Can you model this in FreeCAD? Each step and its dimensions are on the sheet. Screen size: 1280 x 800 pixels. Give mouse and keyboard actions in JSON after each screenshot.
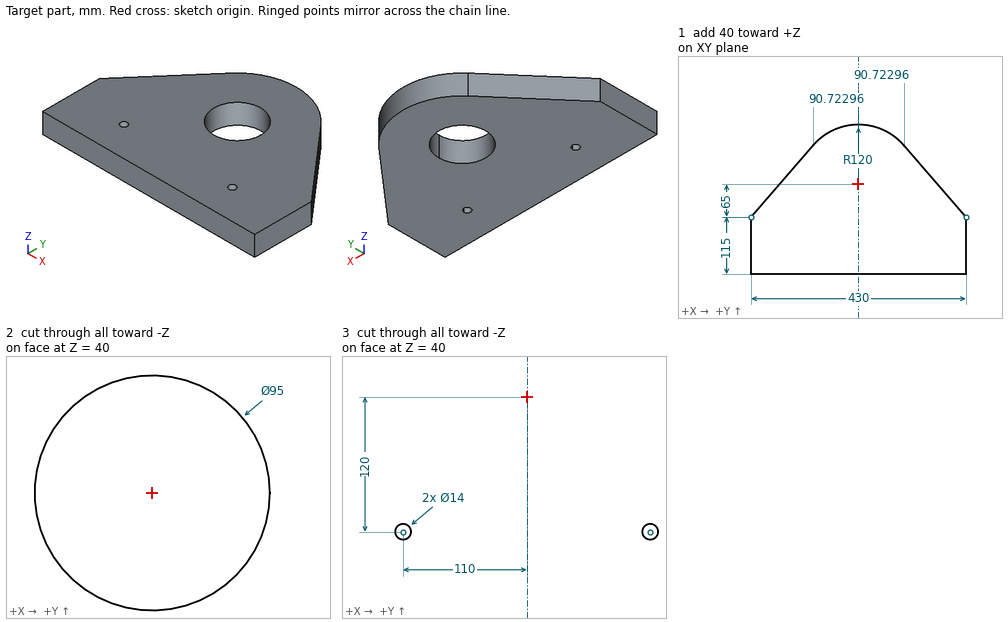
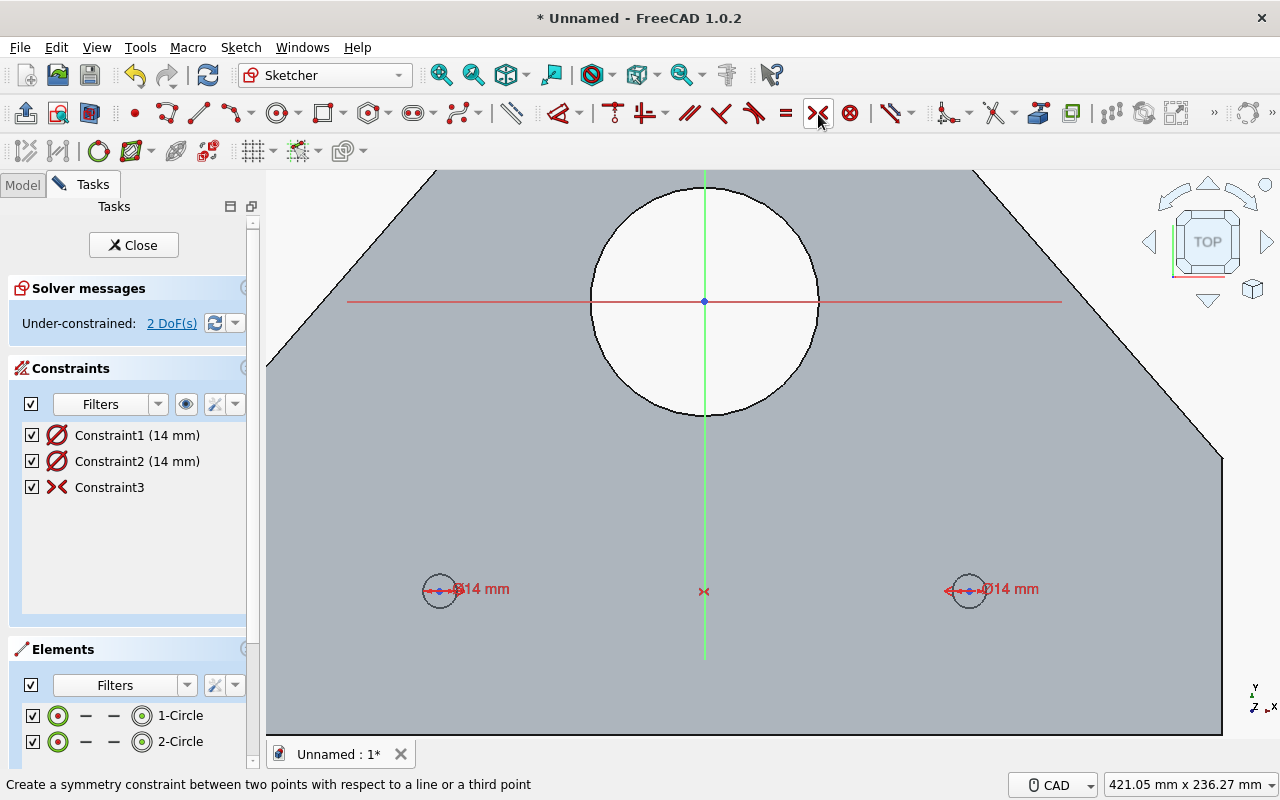
{"action": "left_click", "coordinate": [558, 114]}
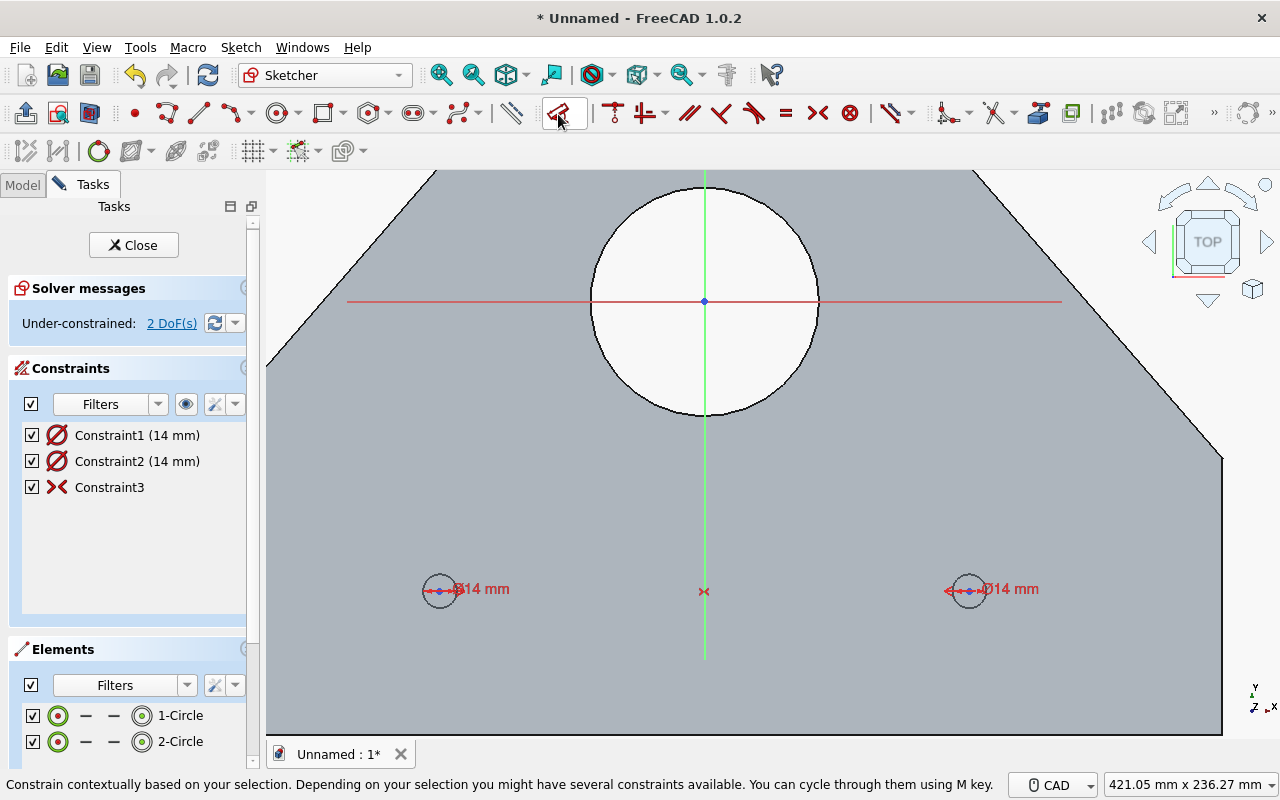
{"action": "left_click", "coordinate": [440, 591]}
{"action": "left_click", "coordinate": [572, 268]}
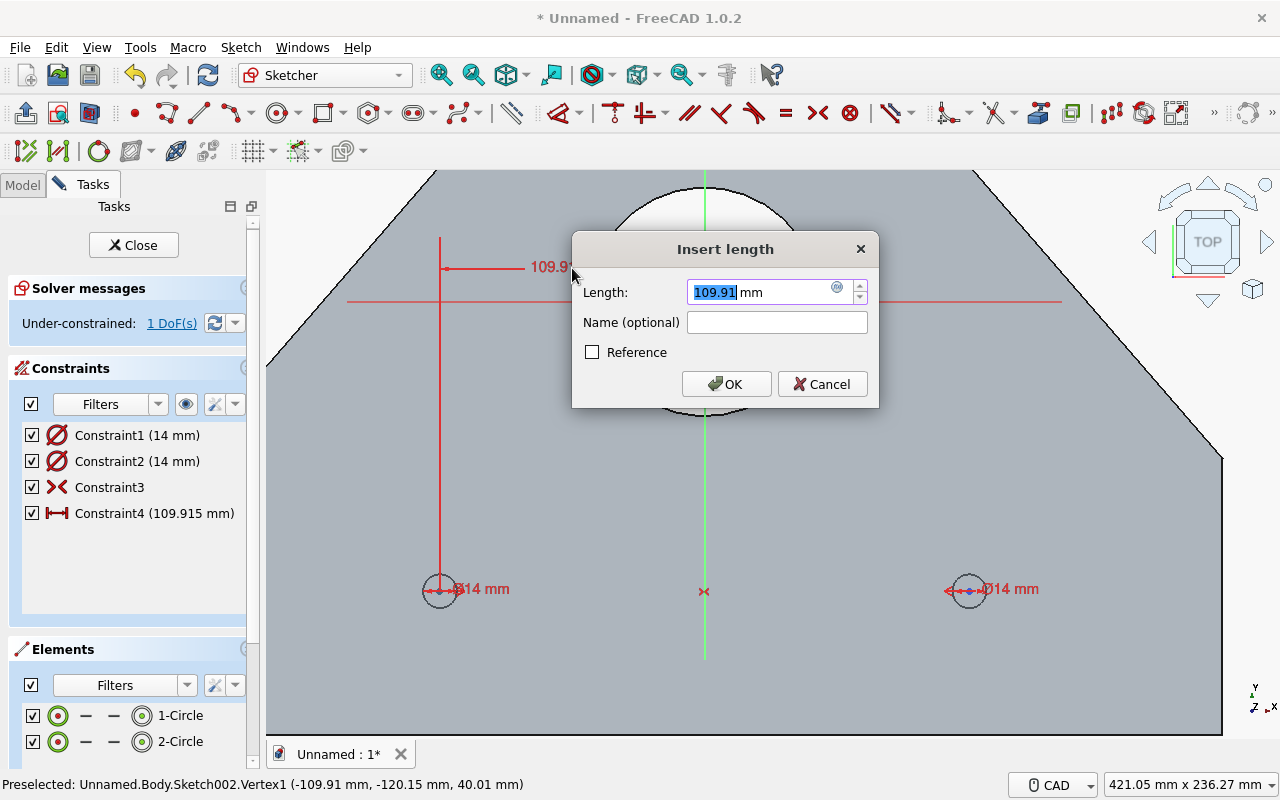
{"action": "type", "text": "110"}
{"action": "key", "text": "Return"}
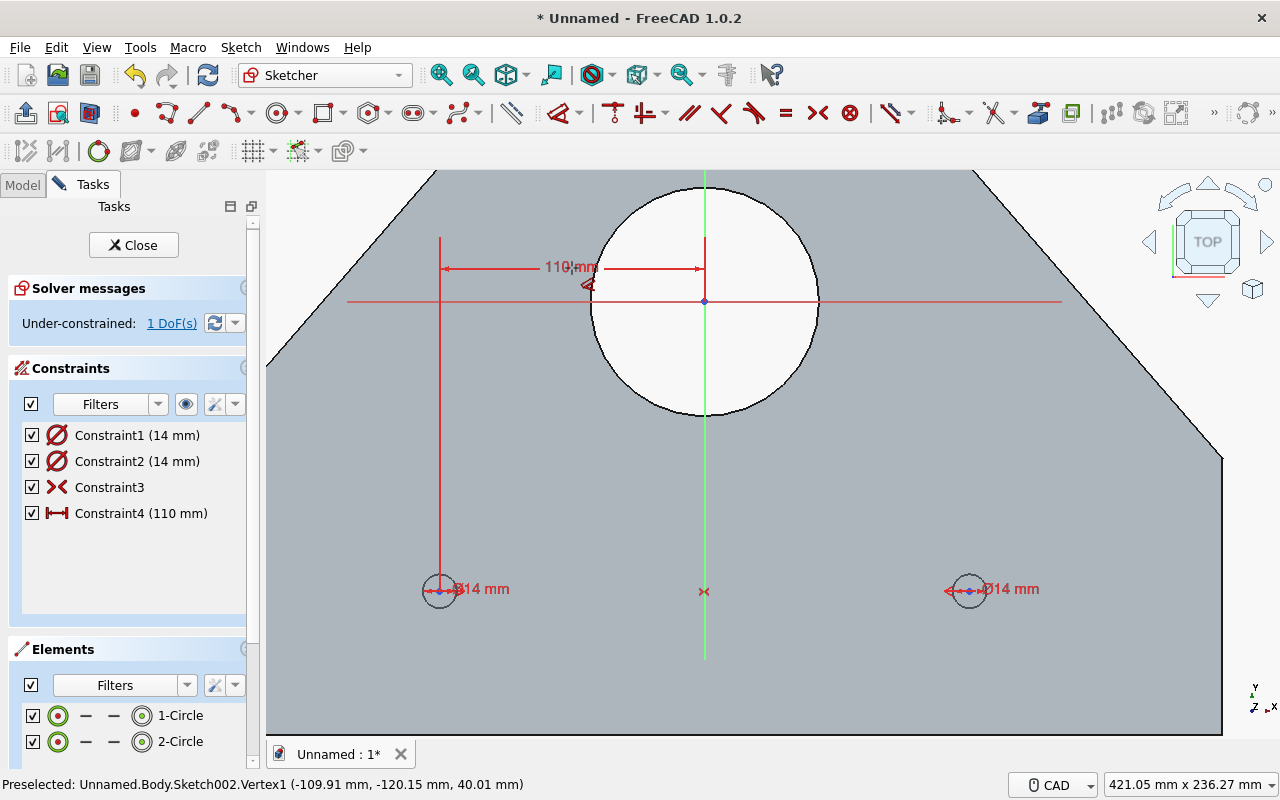
{"action": "left_click", "coordinate": [440, 591]}
{"action": "left_click", "coordinate": [406, 447]}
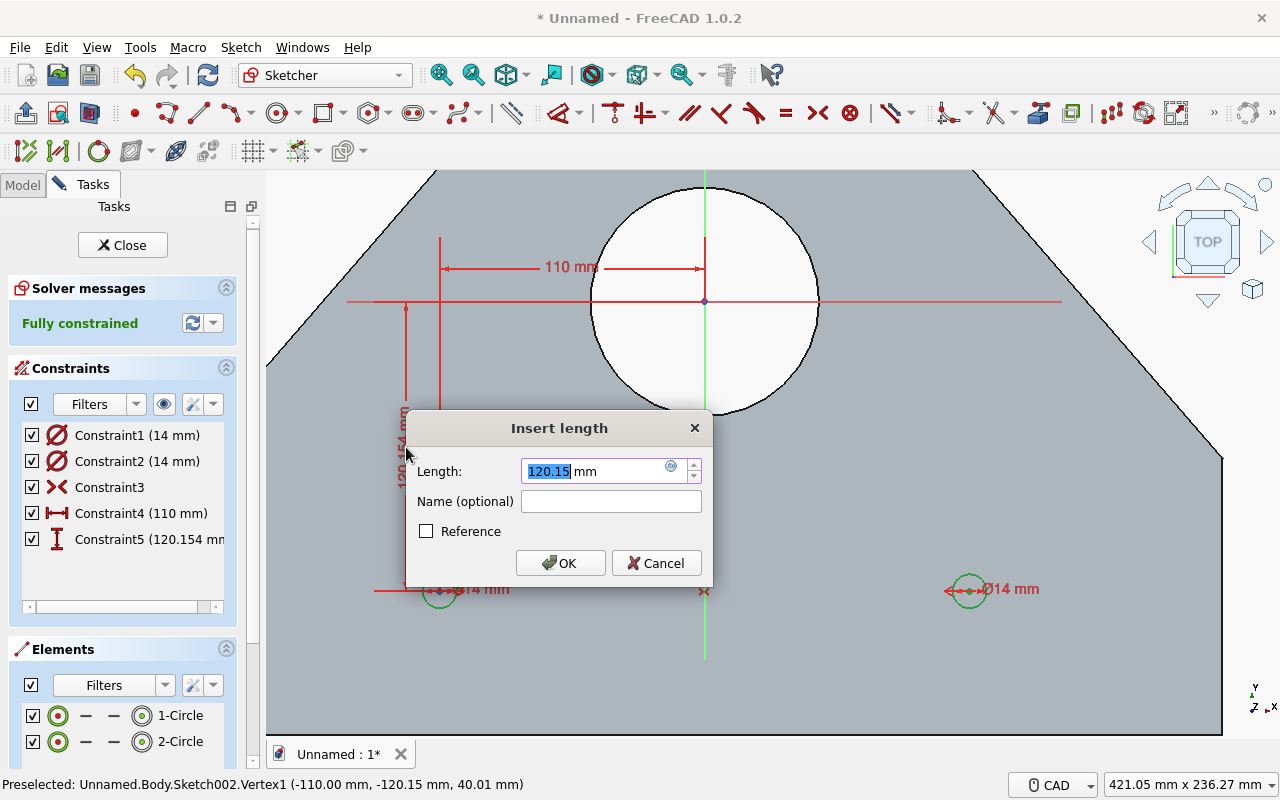
{"action": "type", "text": "120"}
{"action": "key", "text": "Return"}
{"action": "key", "text": "Escape"}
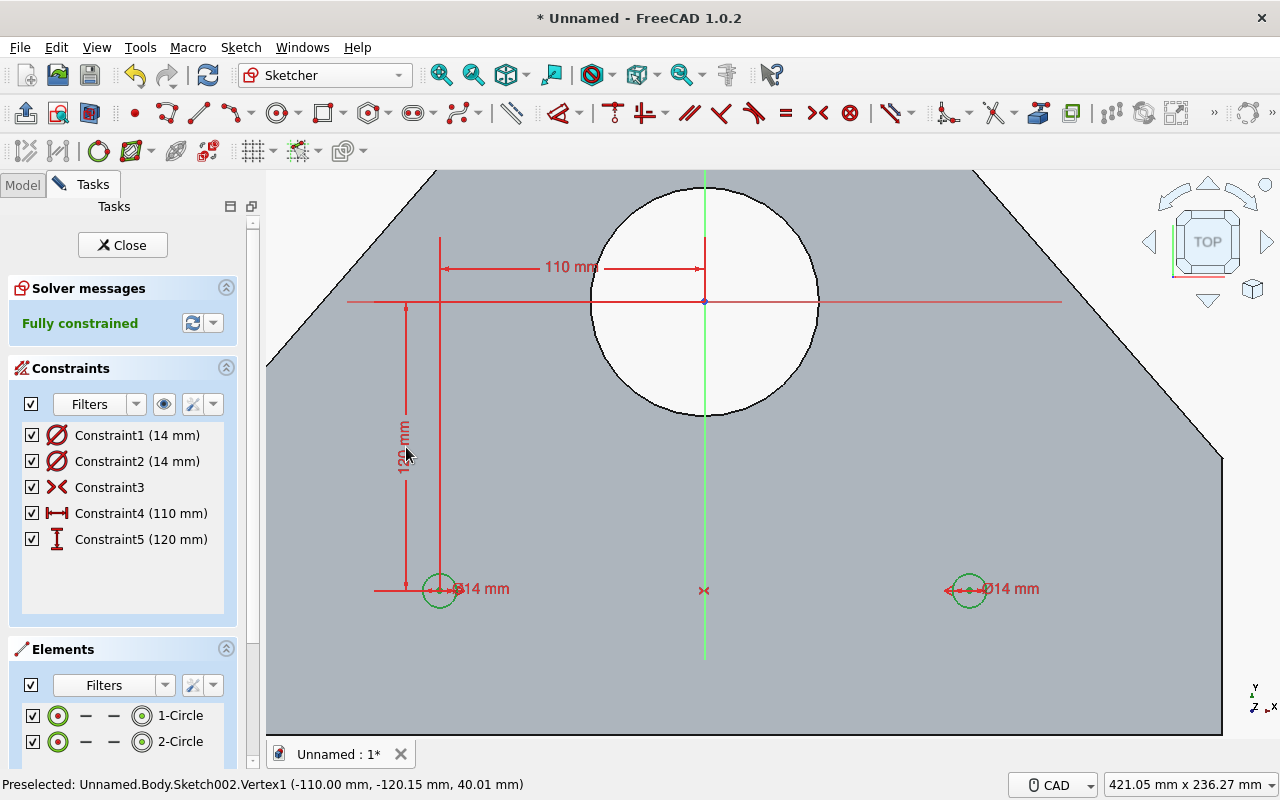
{"action": "left_click", "coordinate": [123, 245]}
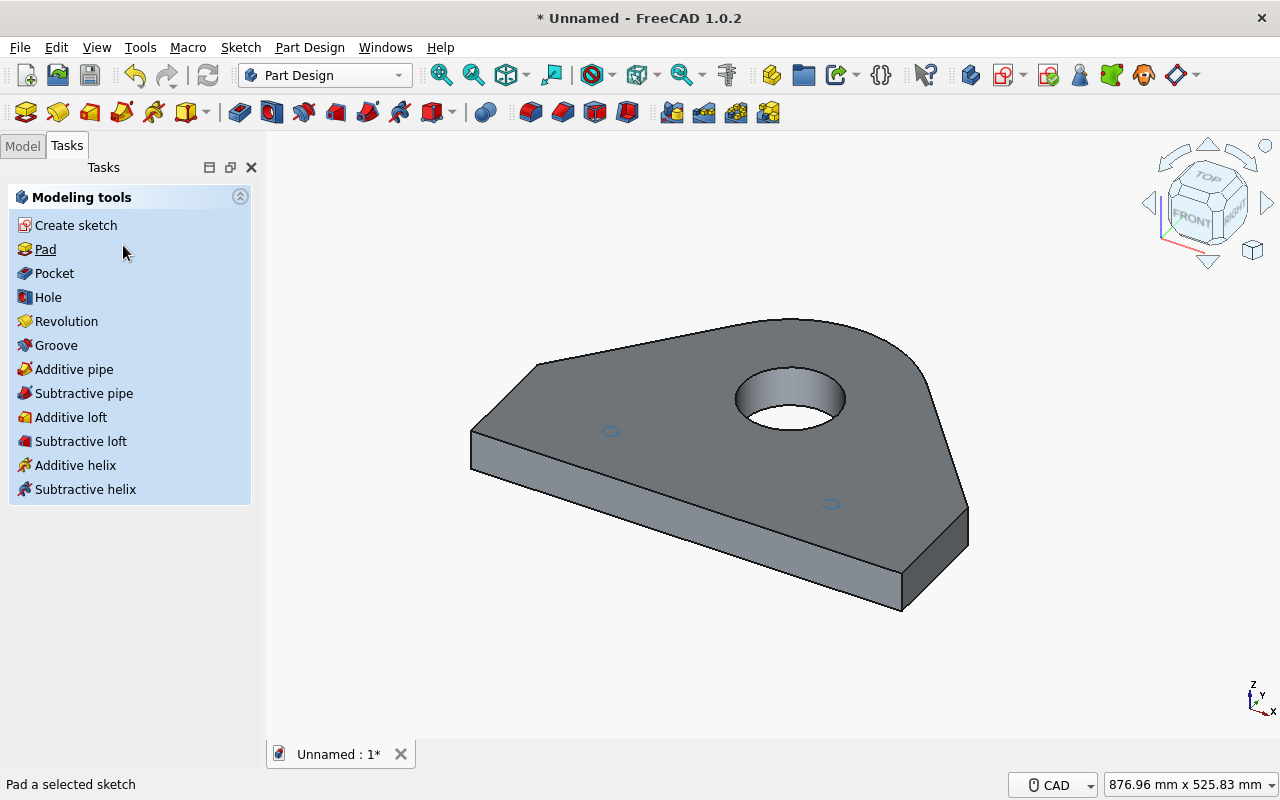
{"action": "left_click", "coordinate": [240, 112]}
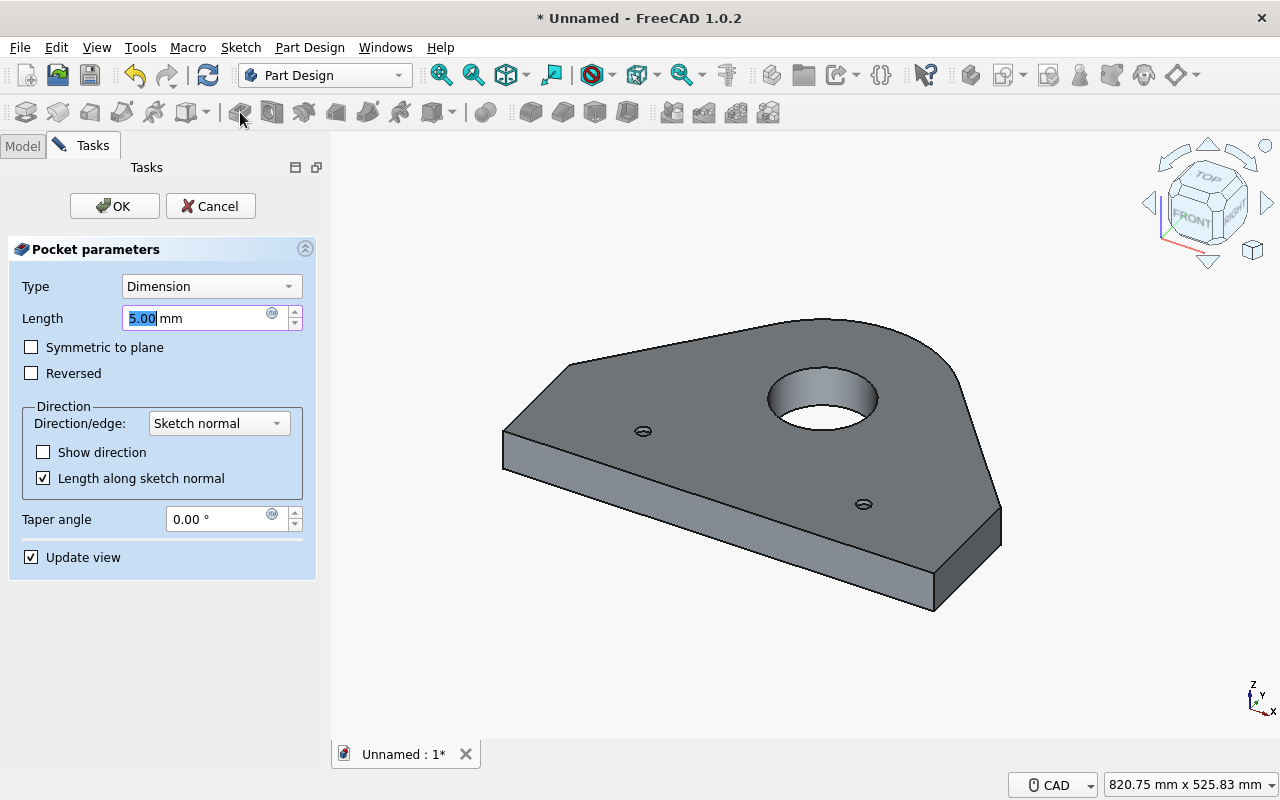
{"action": "left_click", "coordinate": [212, 286]}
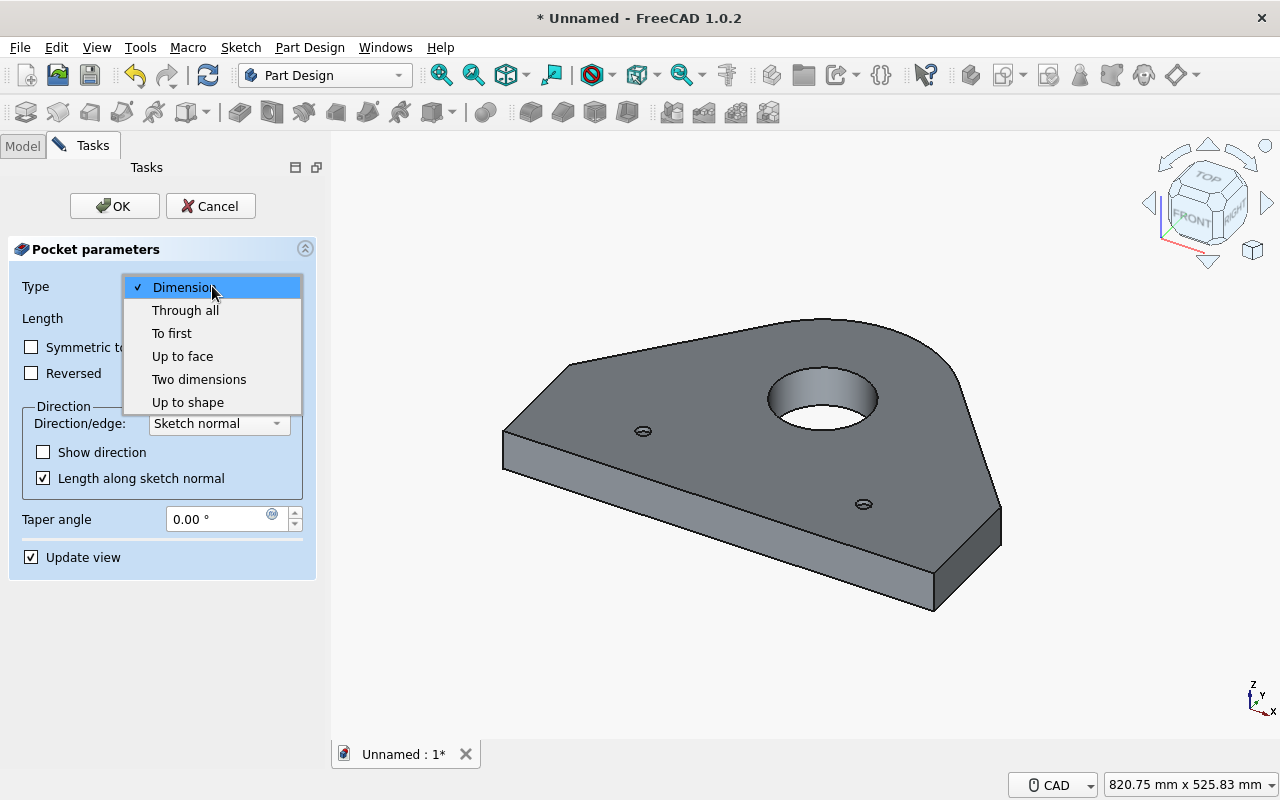
{"action": "left_click", "coordinate": [212, 310]}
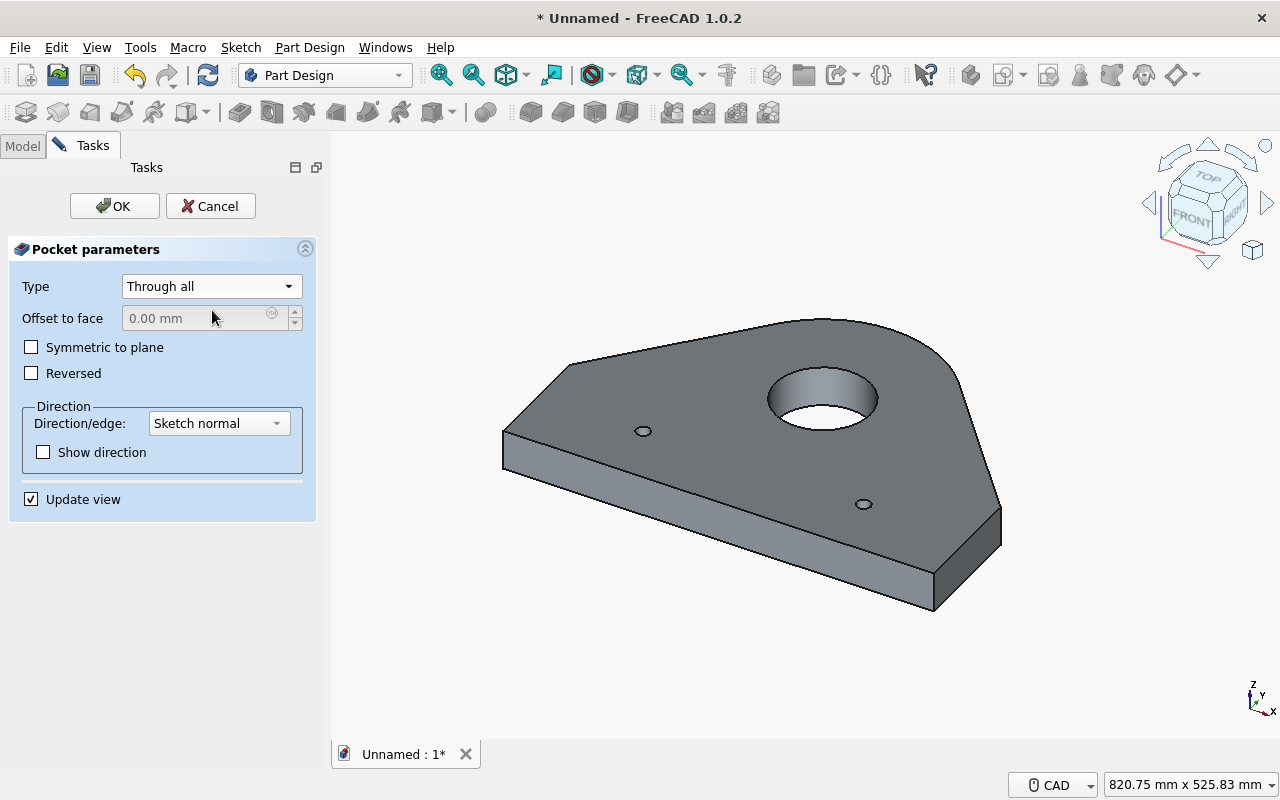
{"action": "left_click", "coordinate": [115, 206]}